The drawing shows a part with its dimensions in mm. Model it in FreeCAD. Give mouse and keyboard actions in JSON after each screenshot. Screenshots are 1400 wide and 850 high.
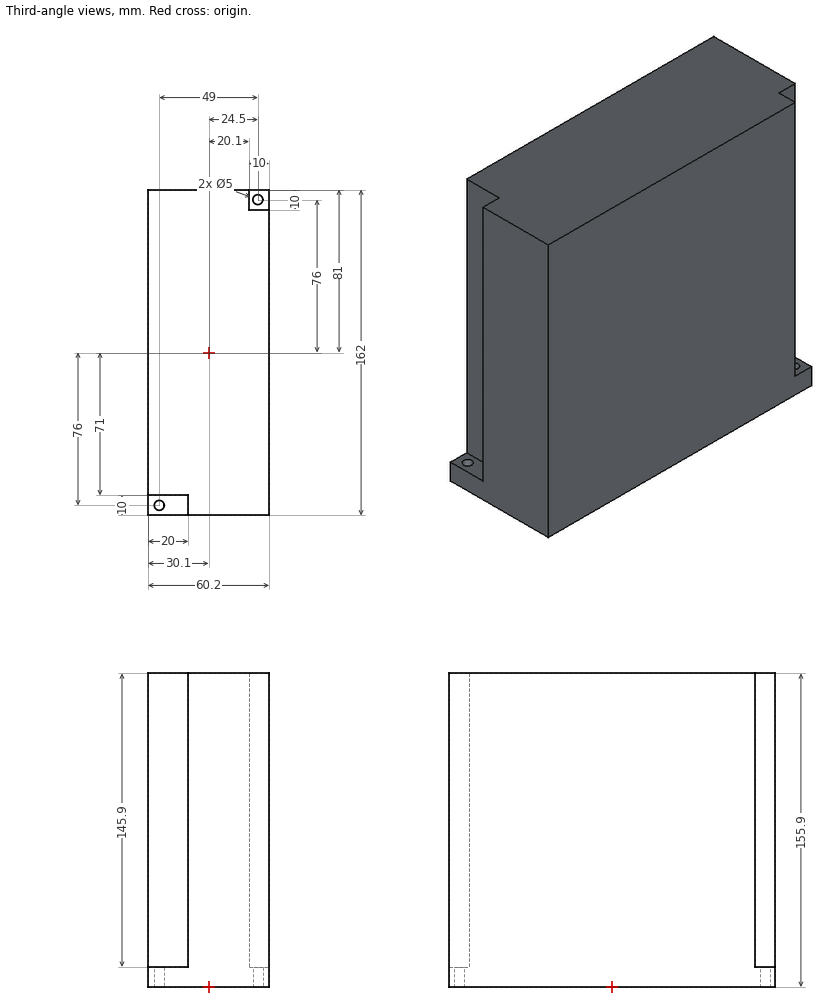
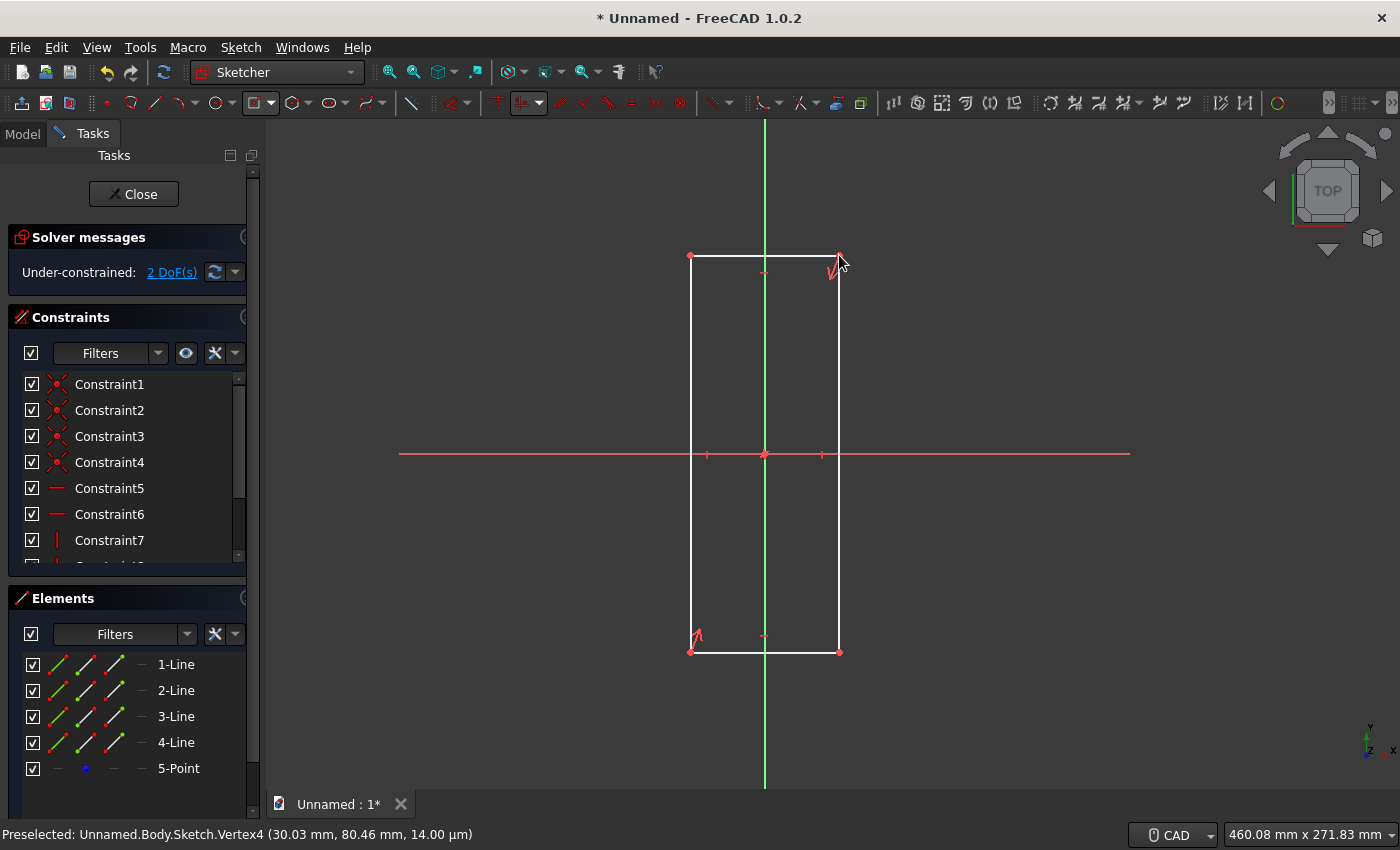
{"action": "left_click", "coordinate": [450, 104]}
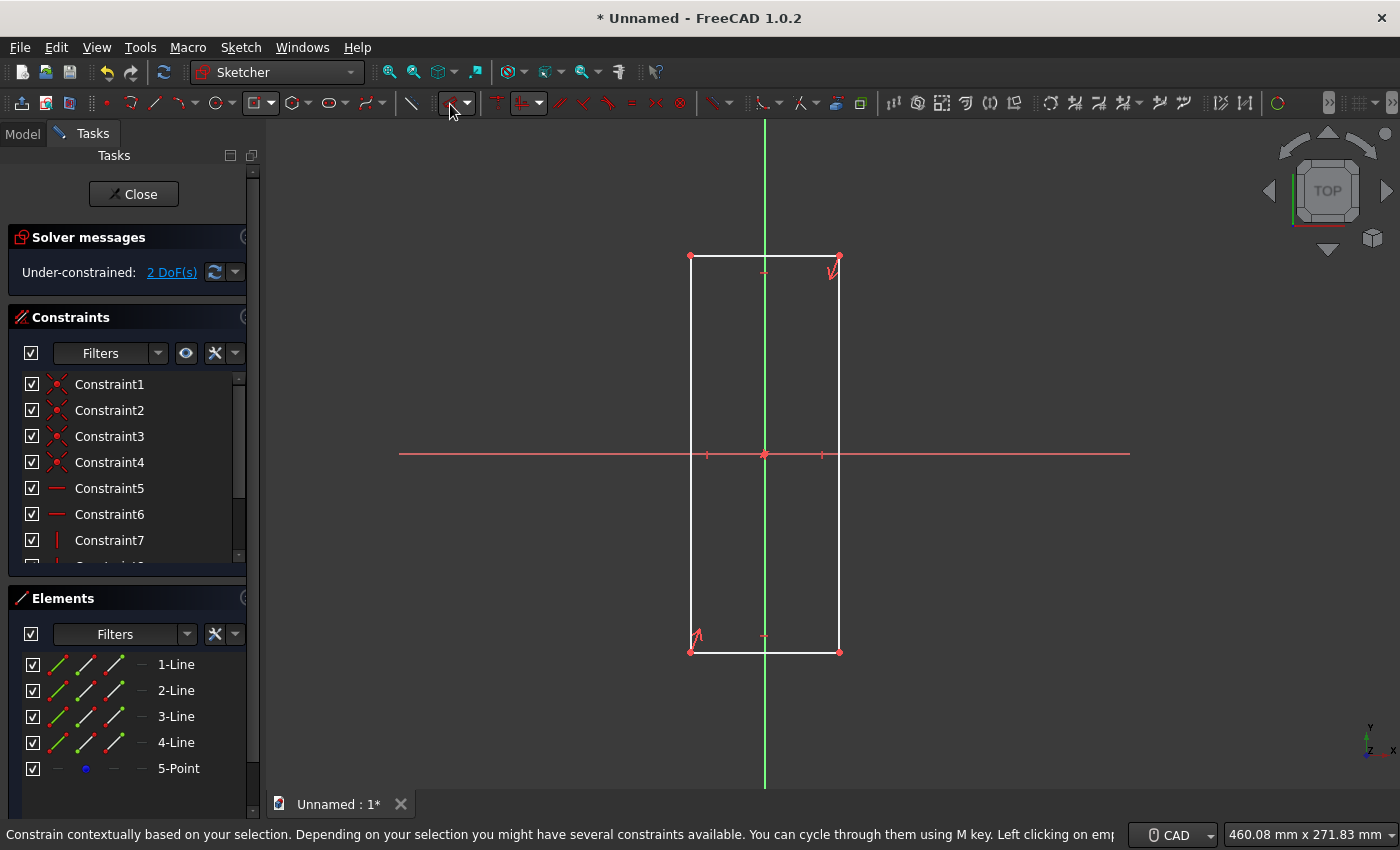
{"action": "left_click", "coordinate": [839, 534]}
{"action": "left_click", "coordinate": [873, 363]}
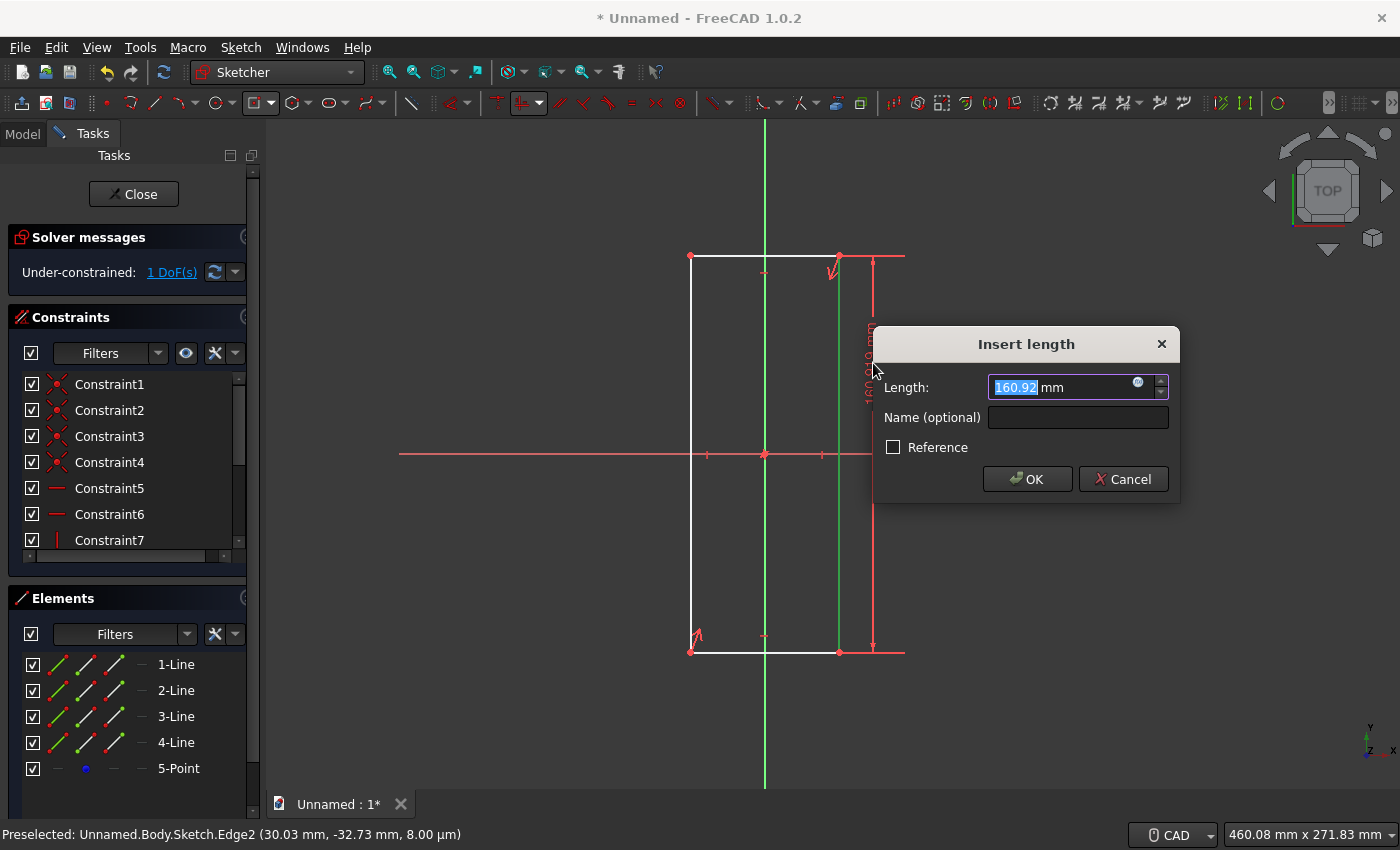
{"action": "type", "text": "162"}
{"action": "key", "text": "Return"}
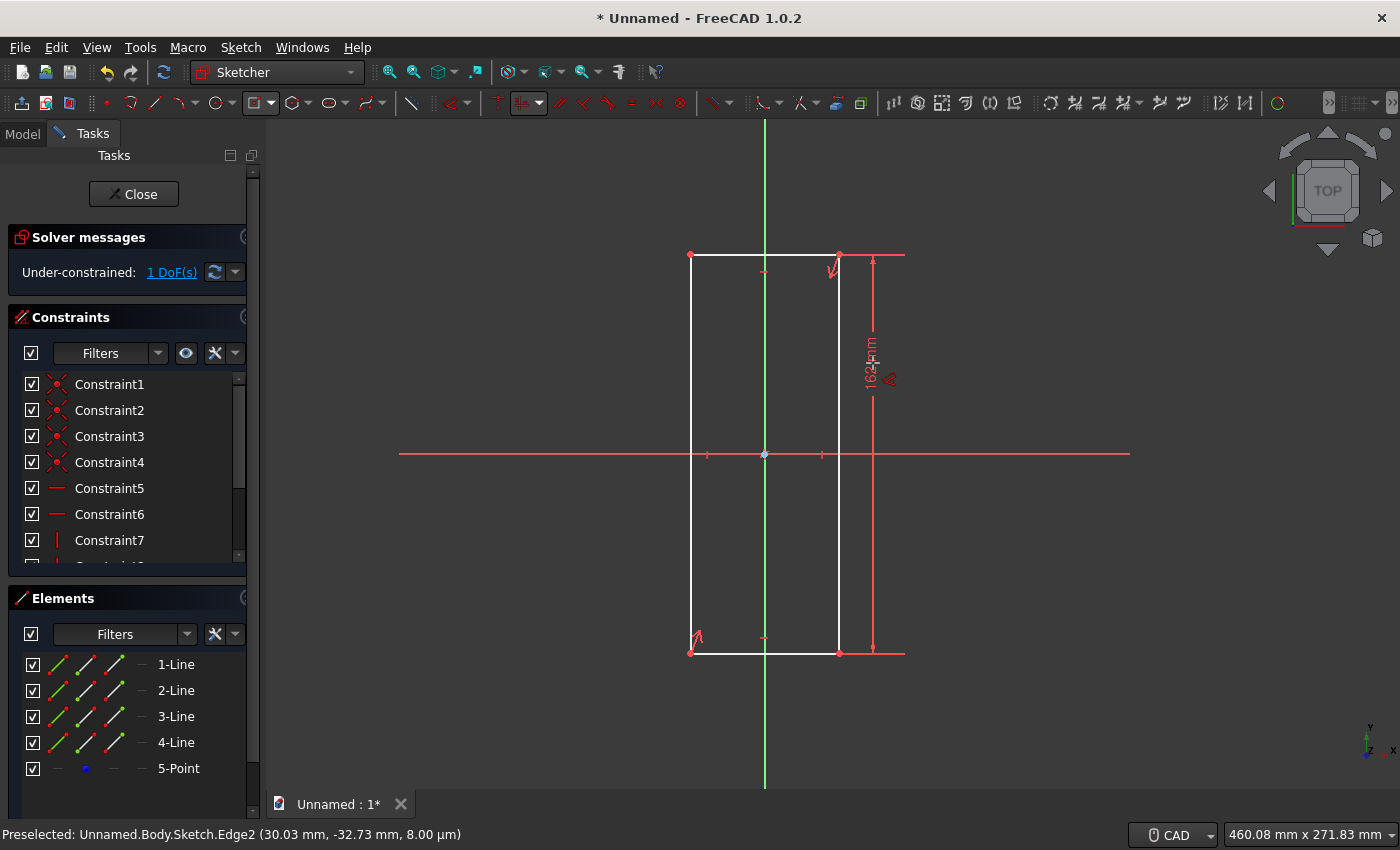
{"action": "left_click", "coordinate": [735, 654]}
{"action": "left_click", "coordinate": [731, 688]}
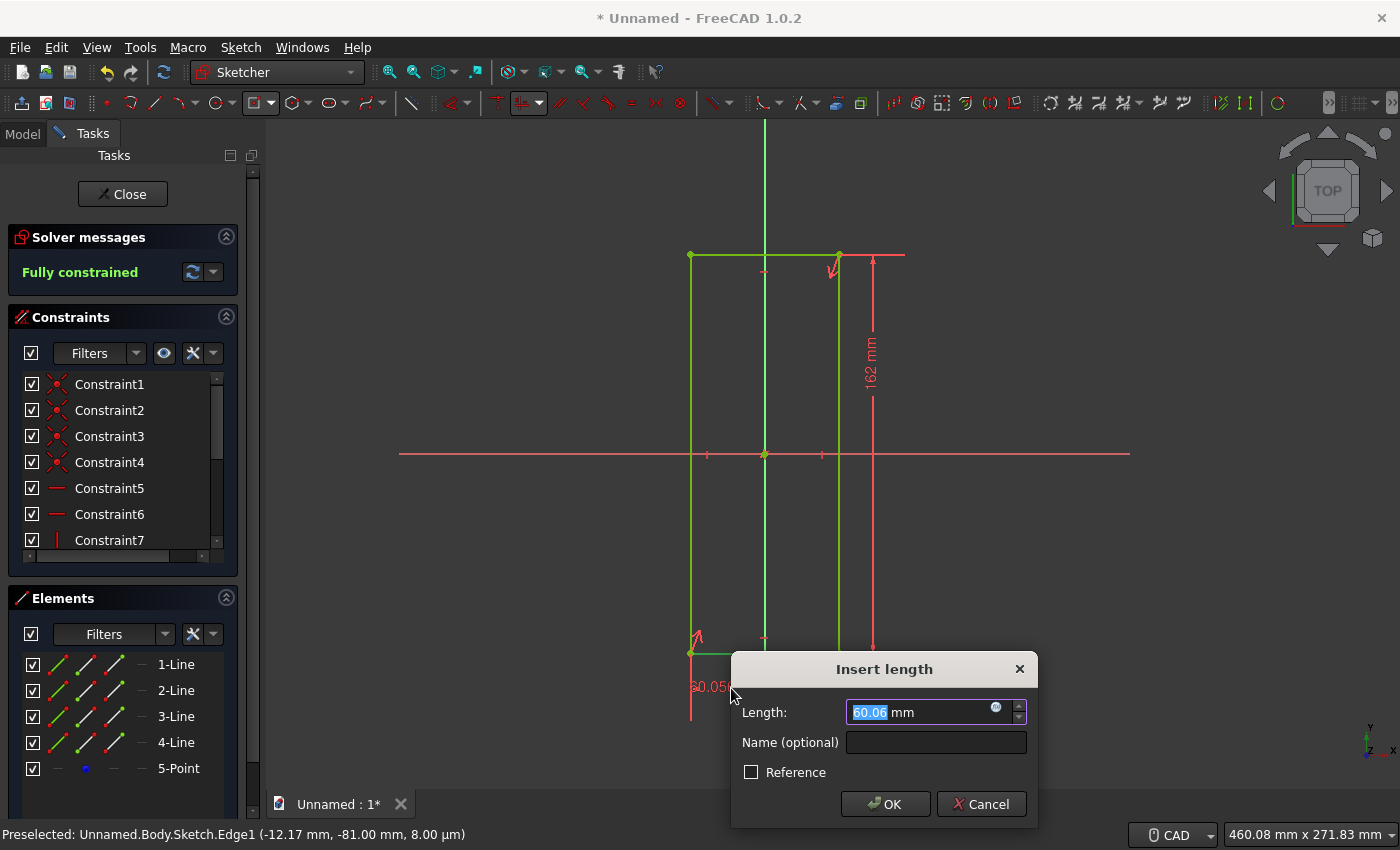
{"action": "type", "text": "60.2"}
{"action": "key", "text": "Return"}
{"action": "key", "text": "Escape"}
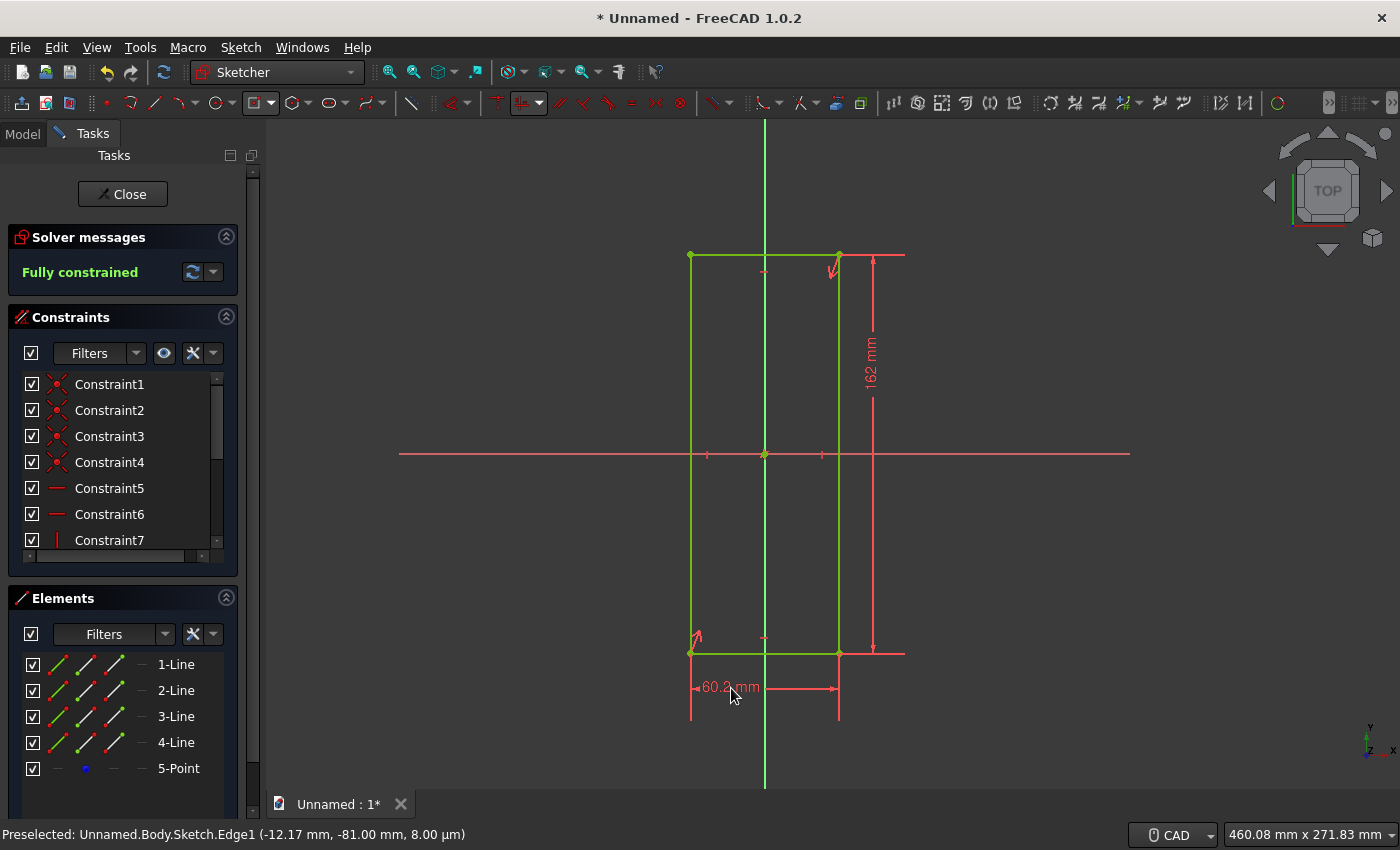
{"action": "left_click", "coordinate": [123, 194]}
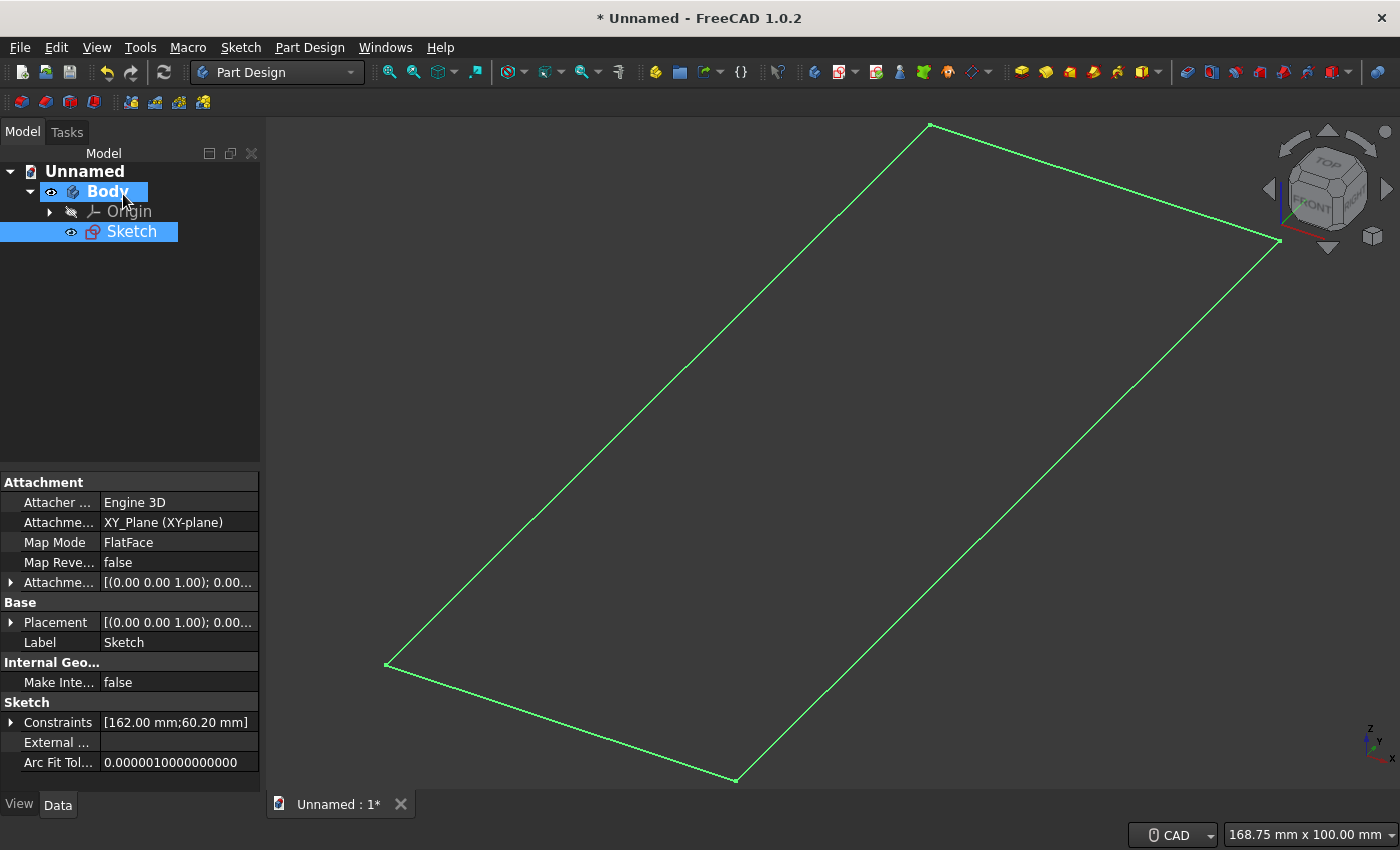
{"action": "left_click", "coordinate": [1022, 72]}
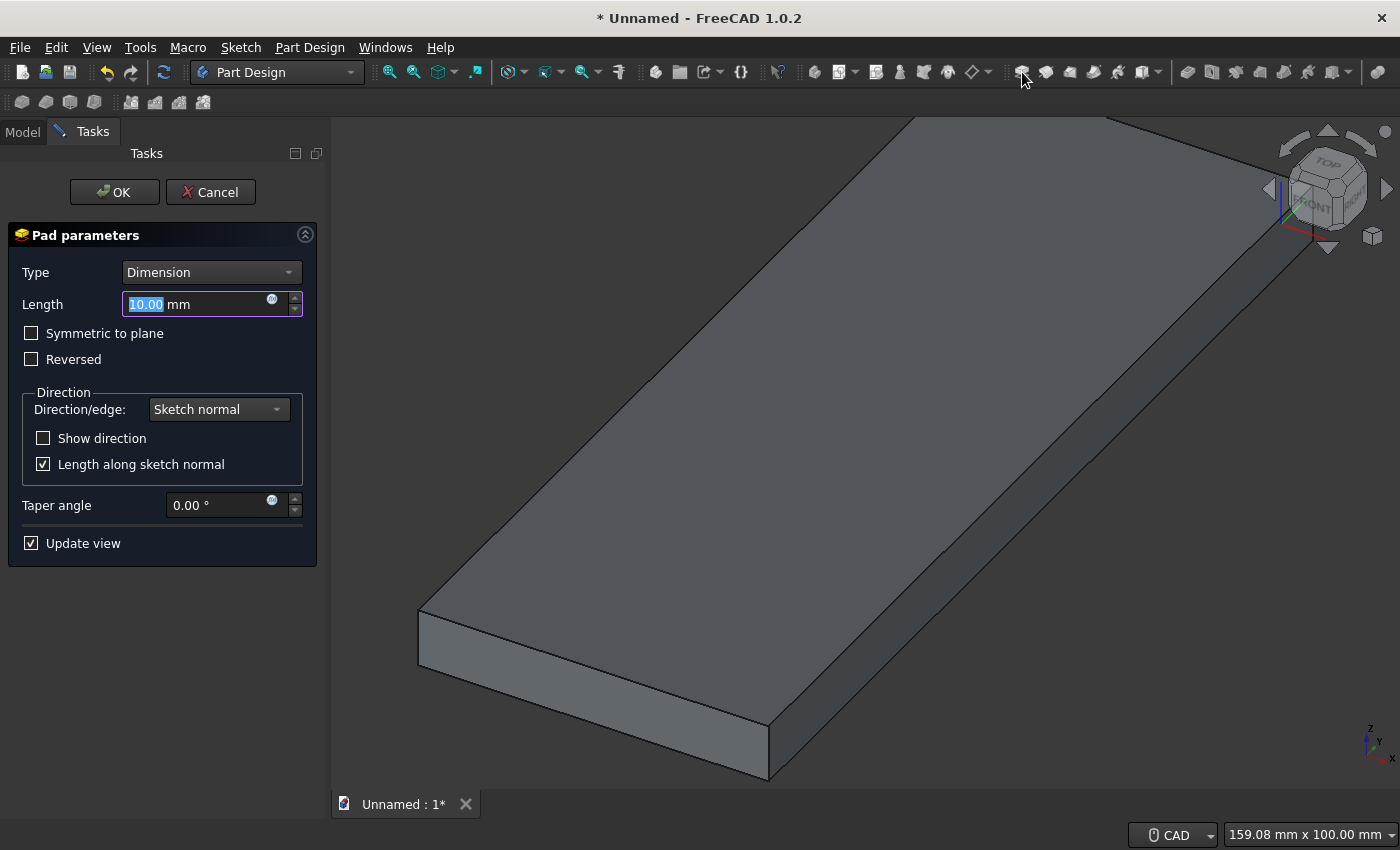
{"action": "type", "text": "155.9"}
{"action": "key", "text": "Tab"}